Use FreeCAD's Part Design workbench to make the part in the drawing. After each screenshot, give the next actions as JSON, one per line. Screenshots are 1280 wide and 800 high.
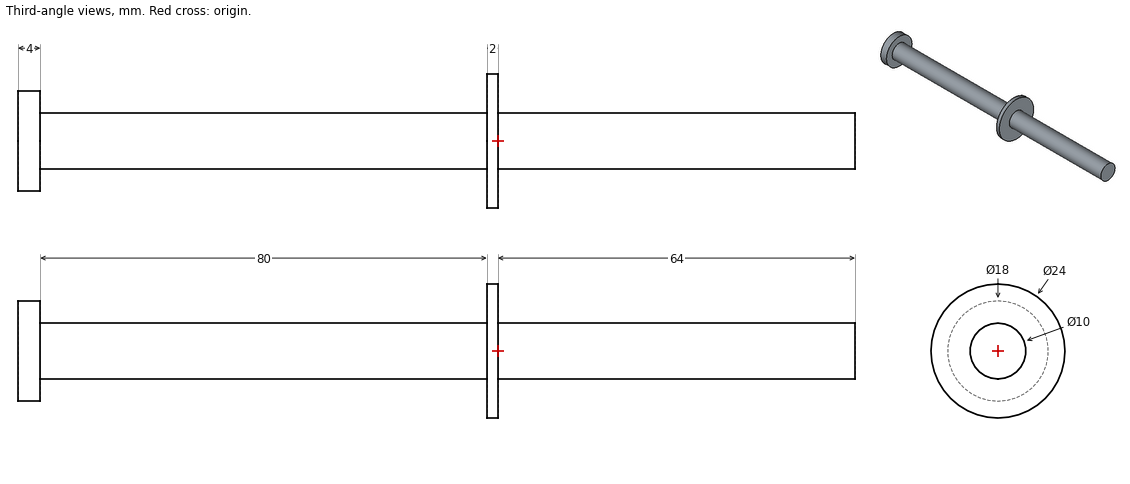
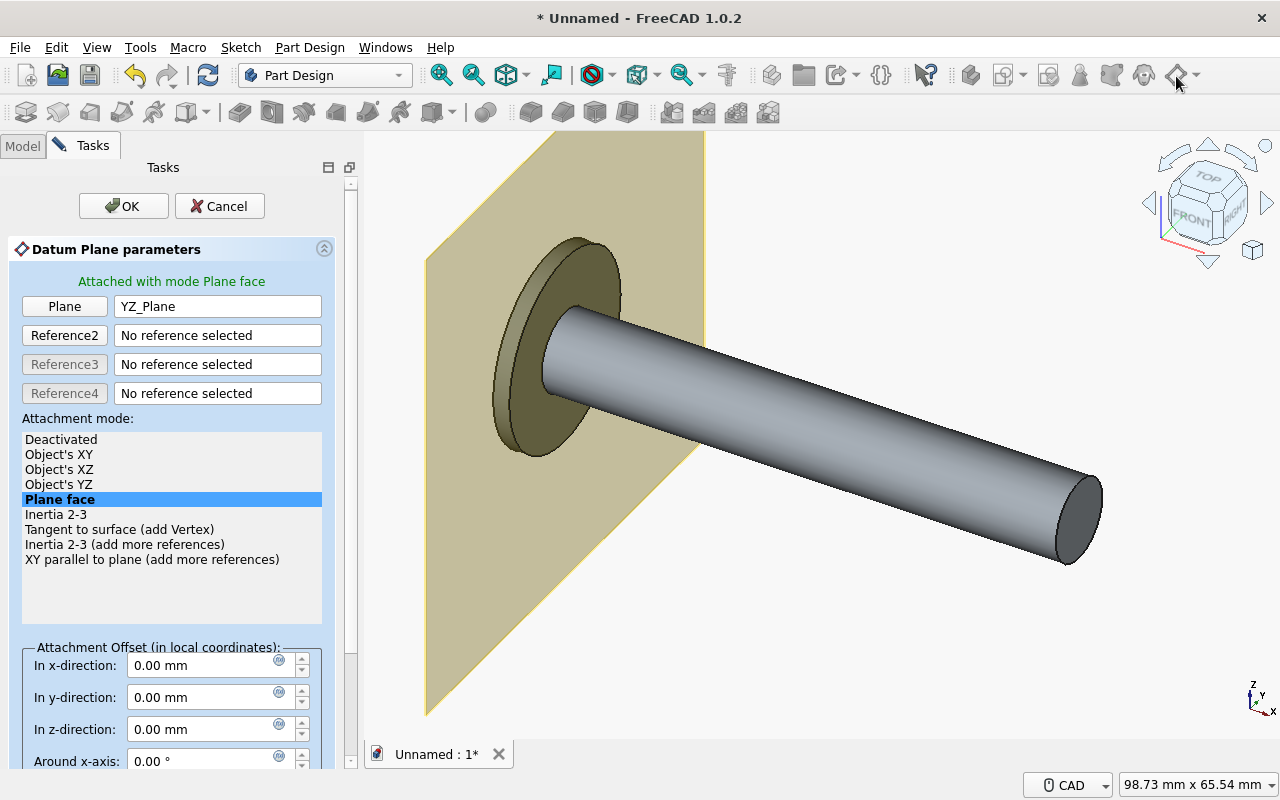
{"action": "triple_click", "coordinate": [210, 729]}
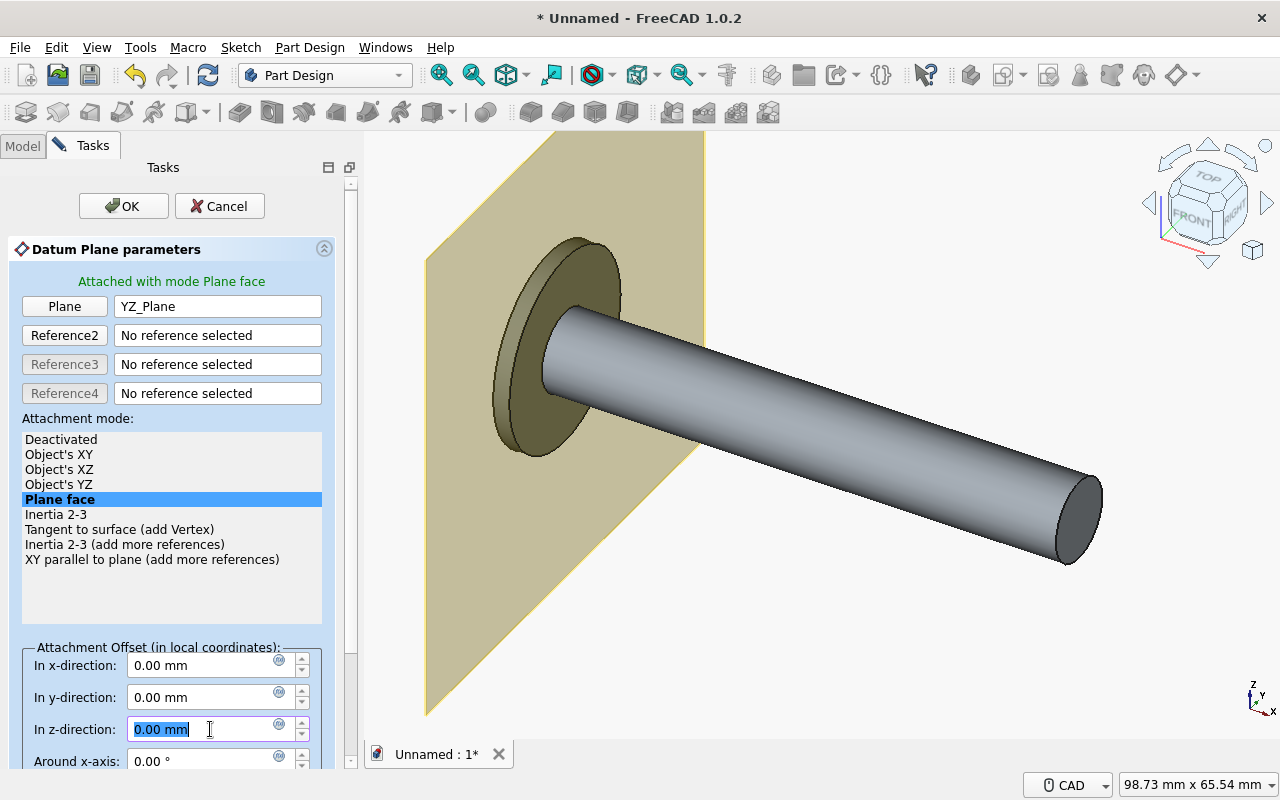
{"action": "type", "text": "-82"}
{"action": "key", "text": "Tab"}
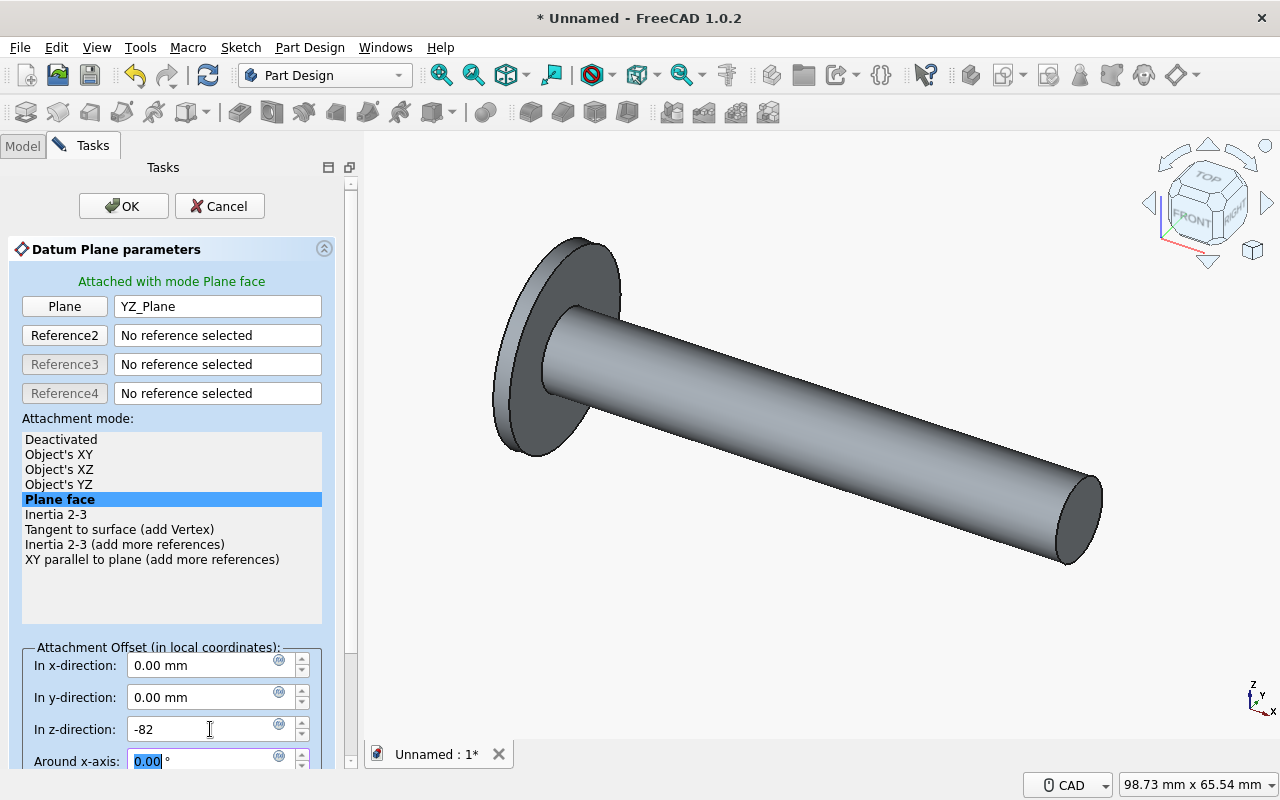
{"action": "left_click", "coordinate": [124, 206]}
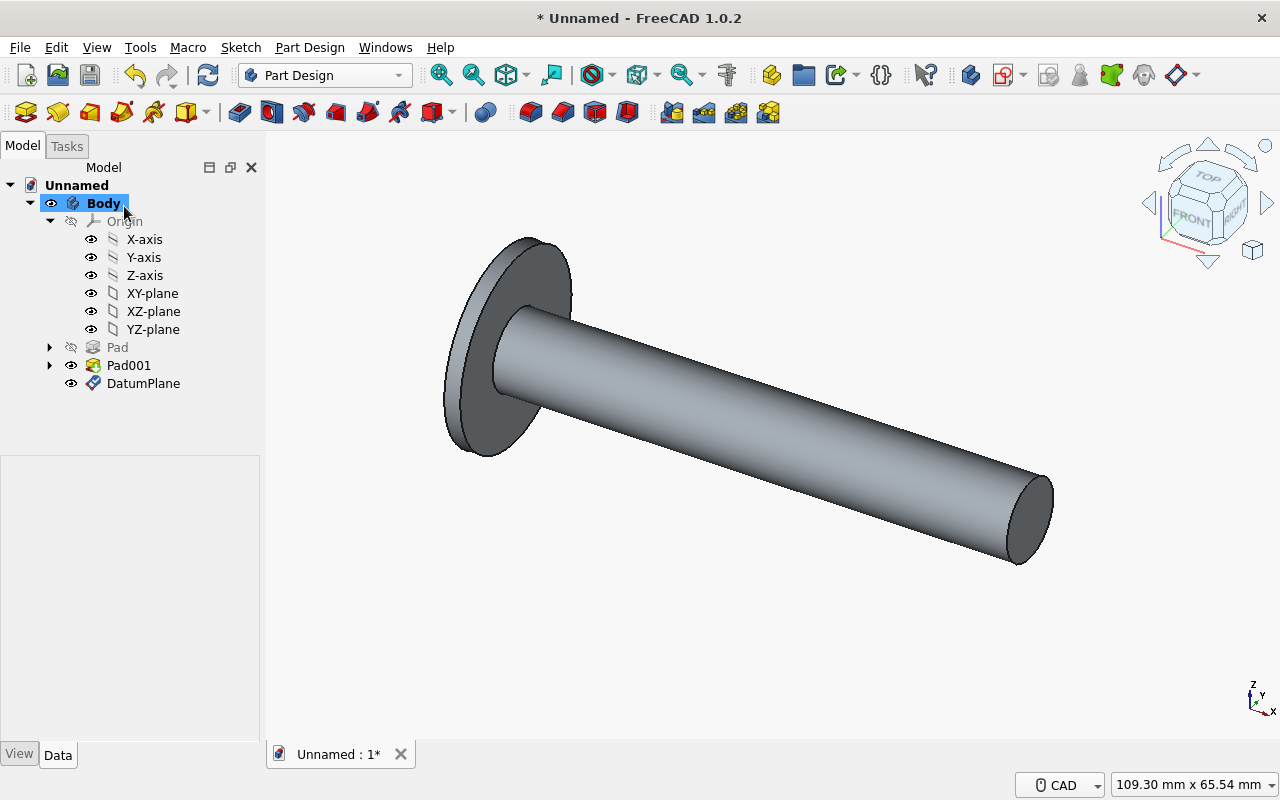
{"action": "left_click", "coordinate": [116, 383]}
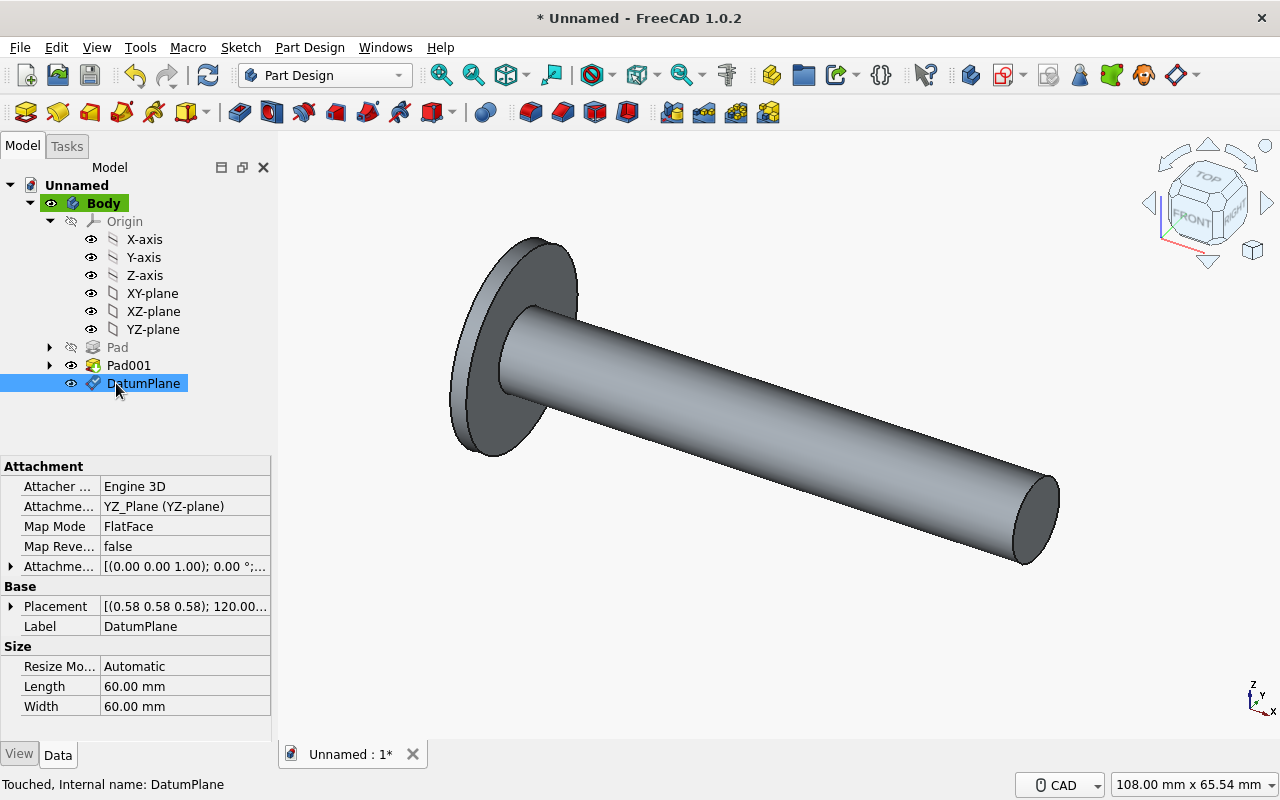
{"action": "left_click", "coordinate": [1004, 76]}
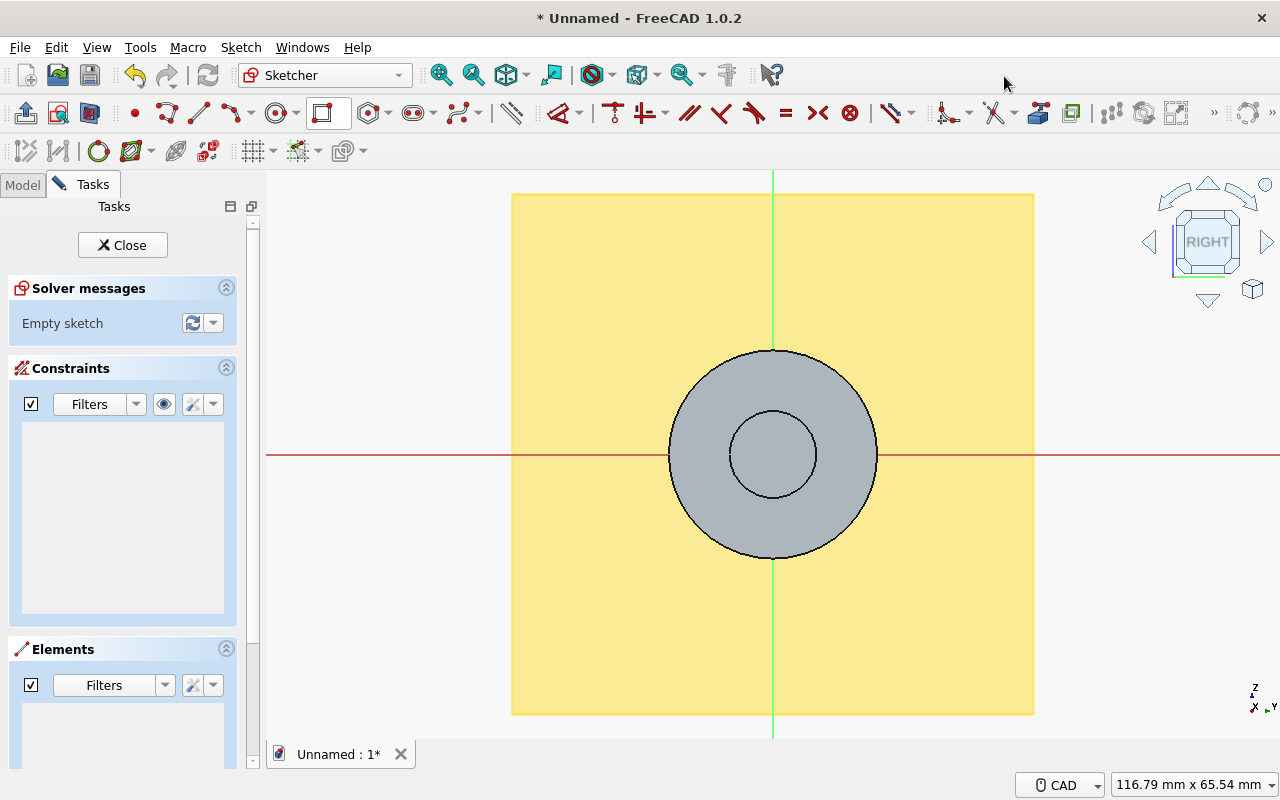
{"action": "key", "text": "q s"}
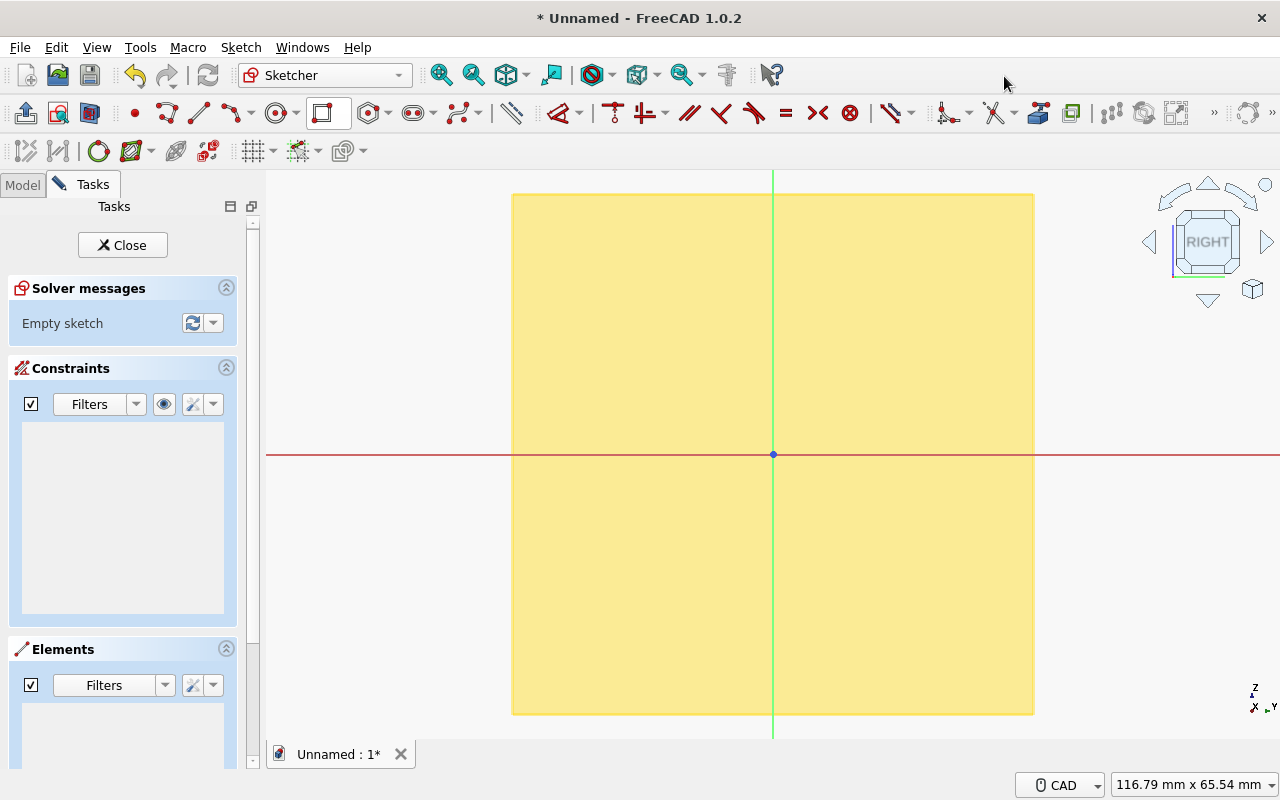
{"action": "scroll", "coordinate": [795, 454], "scroll_direction": "up", "scroll_amount": 7}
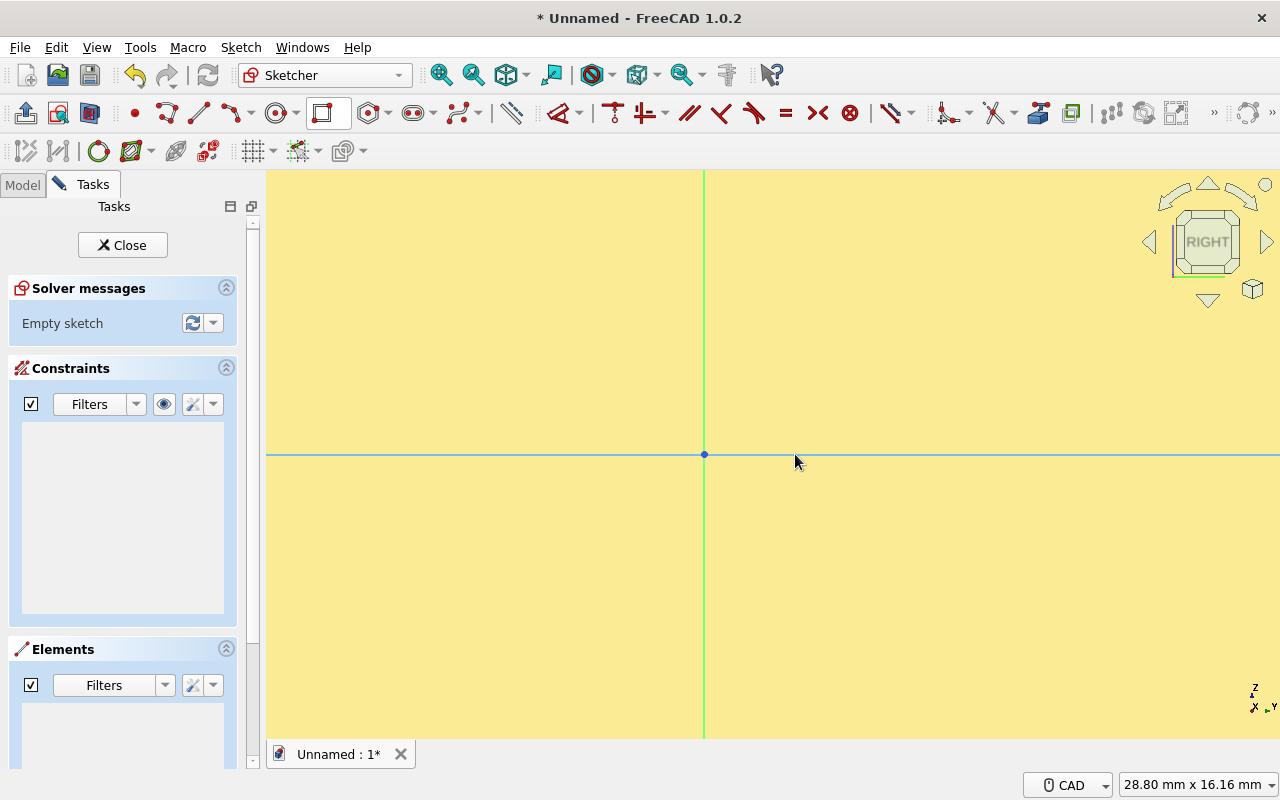
{"action": "key", "text": "g c"}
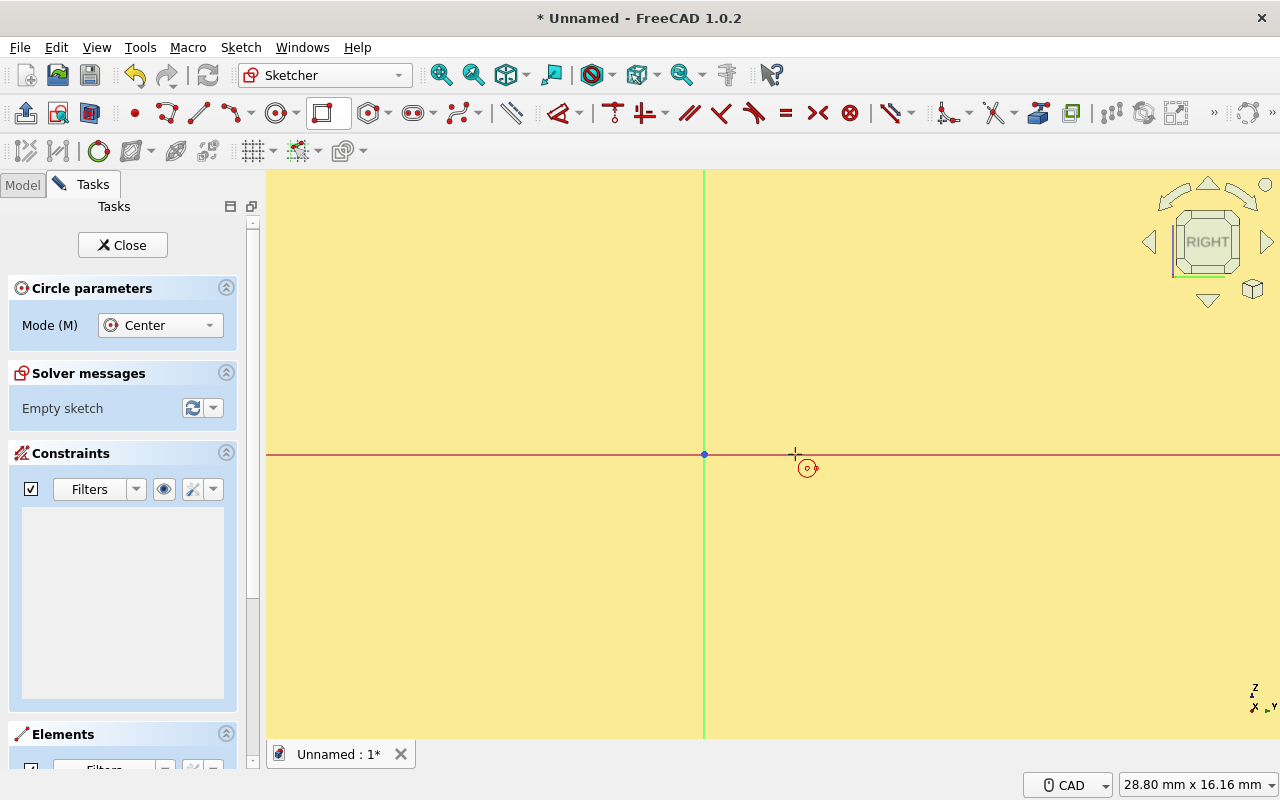
{"action": "left_click", "coordinate": [704, 454]}
{"action": "mouse_move", "coordinate": [829, 330]}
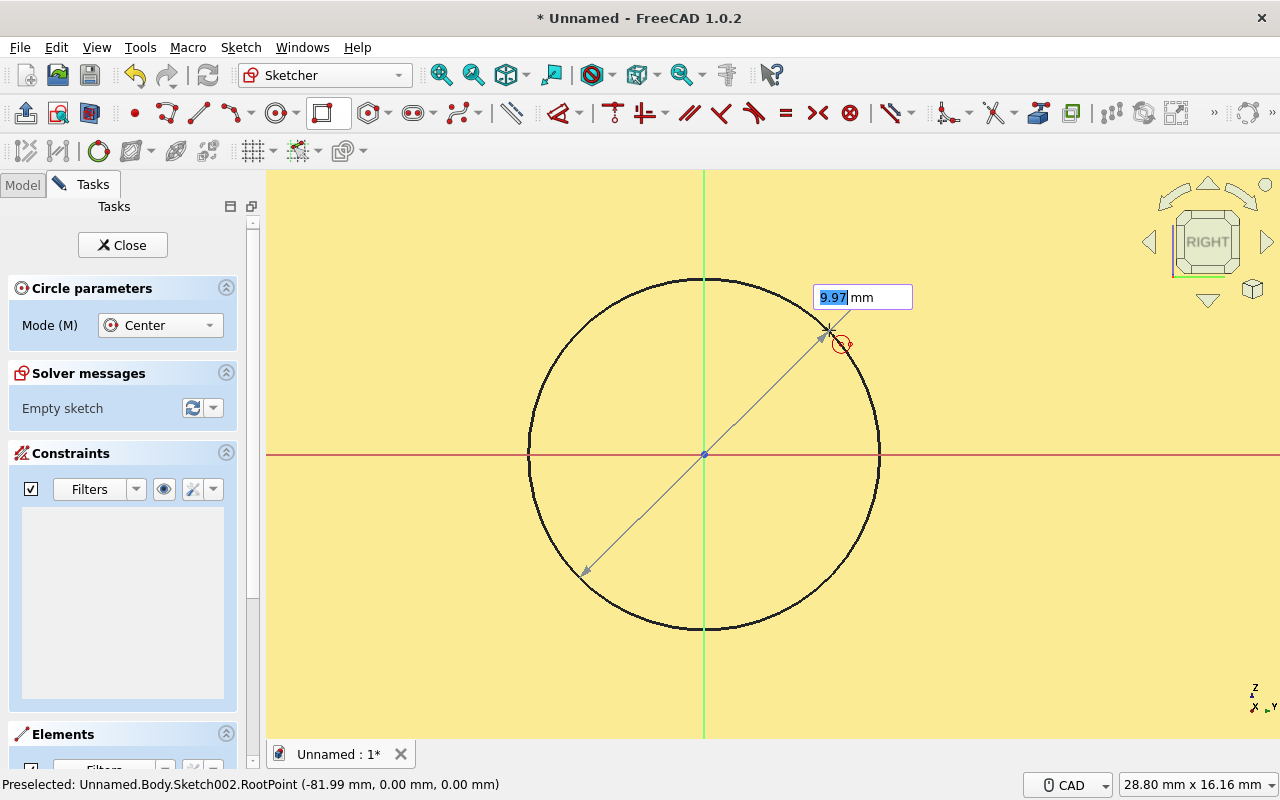
{"action": "type", "text": "10"}
{"action": "key", "text": "Return"}
{"action": "key", "text": "Escape"}